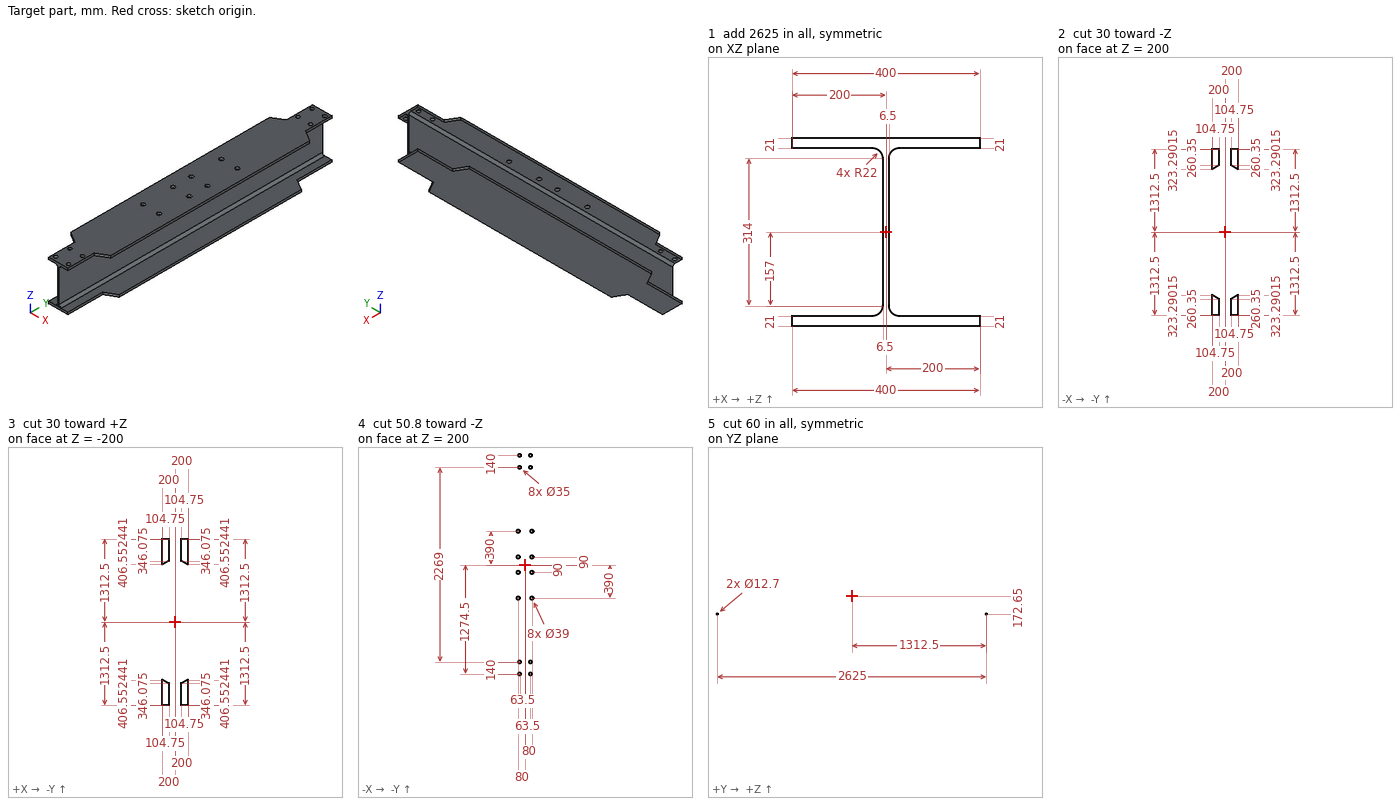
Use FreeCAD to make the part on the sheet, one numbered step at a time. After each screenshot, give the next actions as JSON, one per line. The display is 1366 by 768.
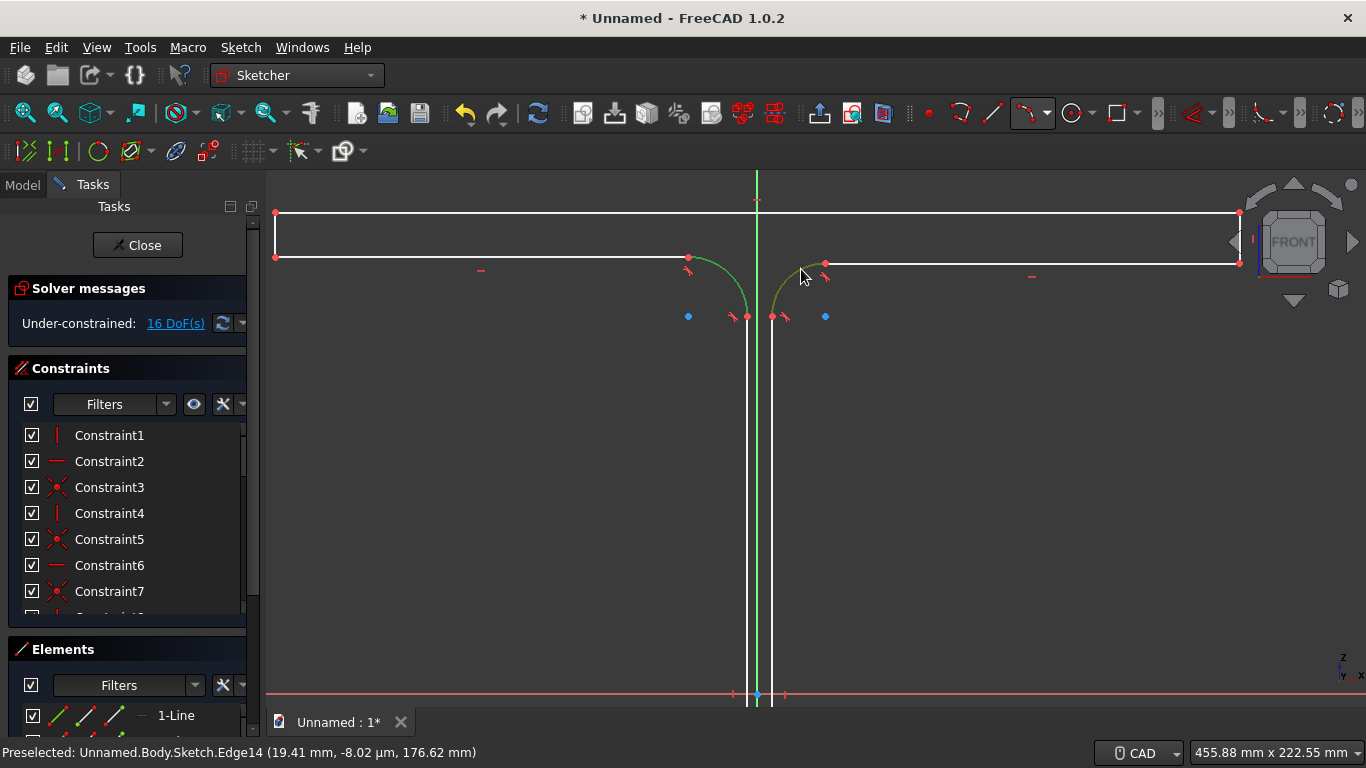
{"action": "scroll", "coordinate": [742, 290], "scroll_direction": "down", "scroll_amount": 5}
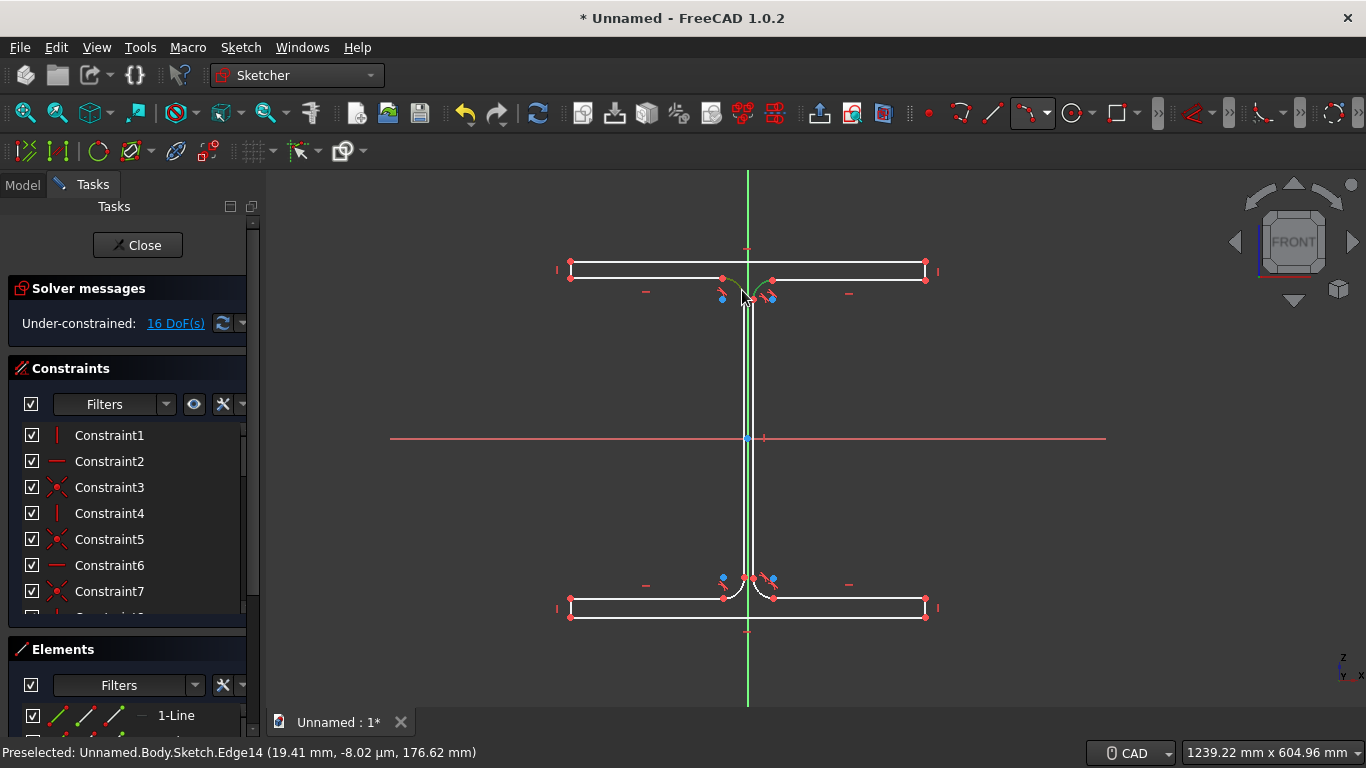
{"action": "scroll", "coordinate": [756, 587], "scroll_direction": "up", "scroll_amount": 3}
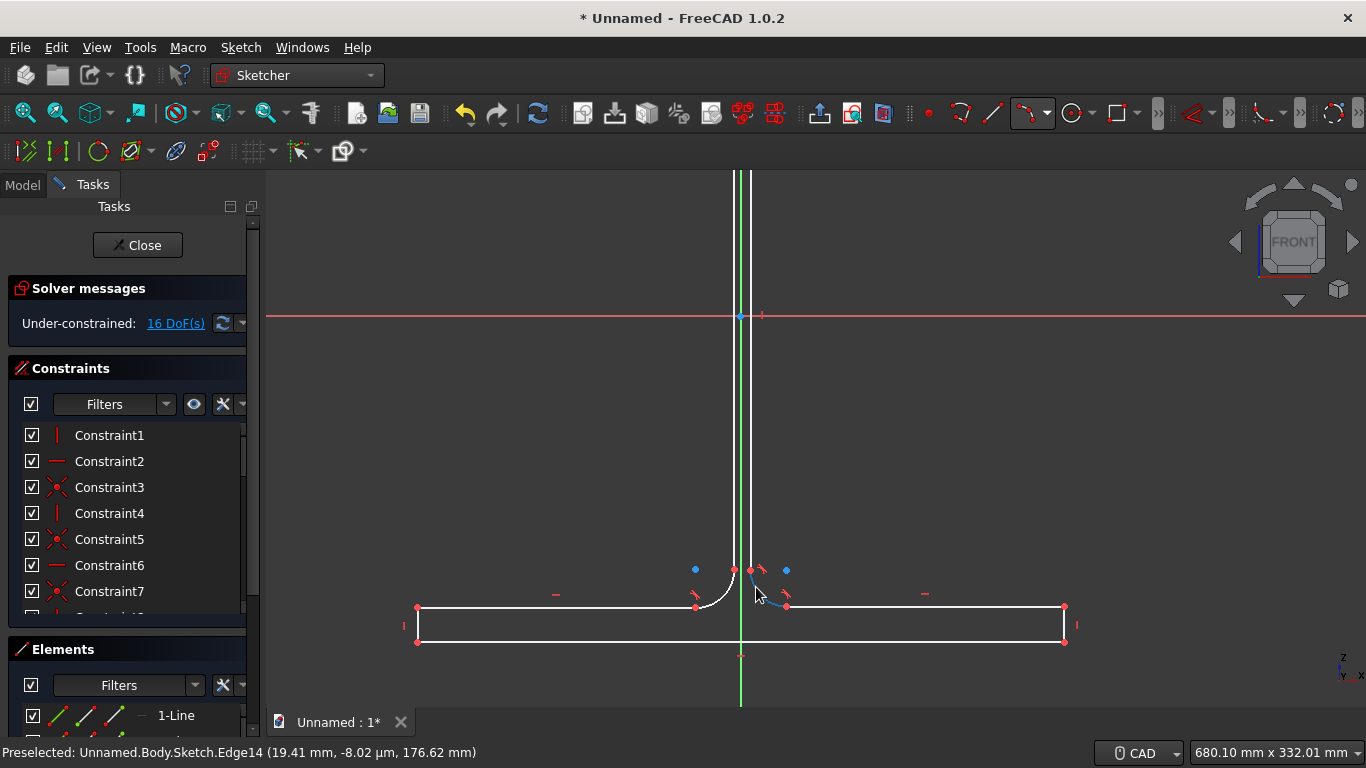
{"action": "left_click", "coordinate": [755, 587]}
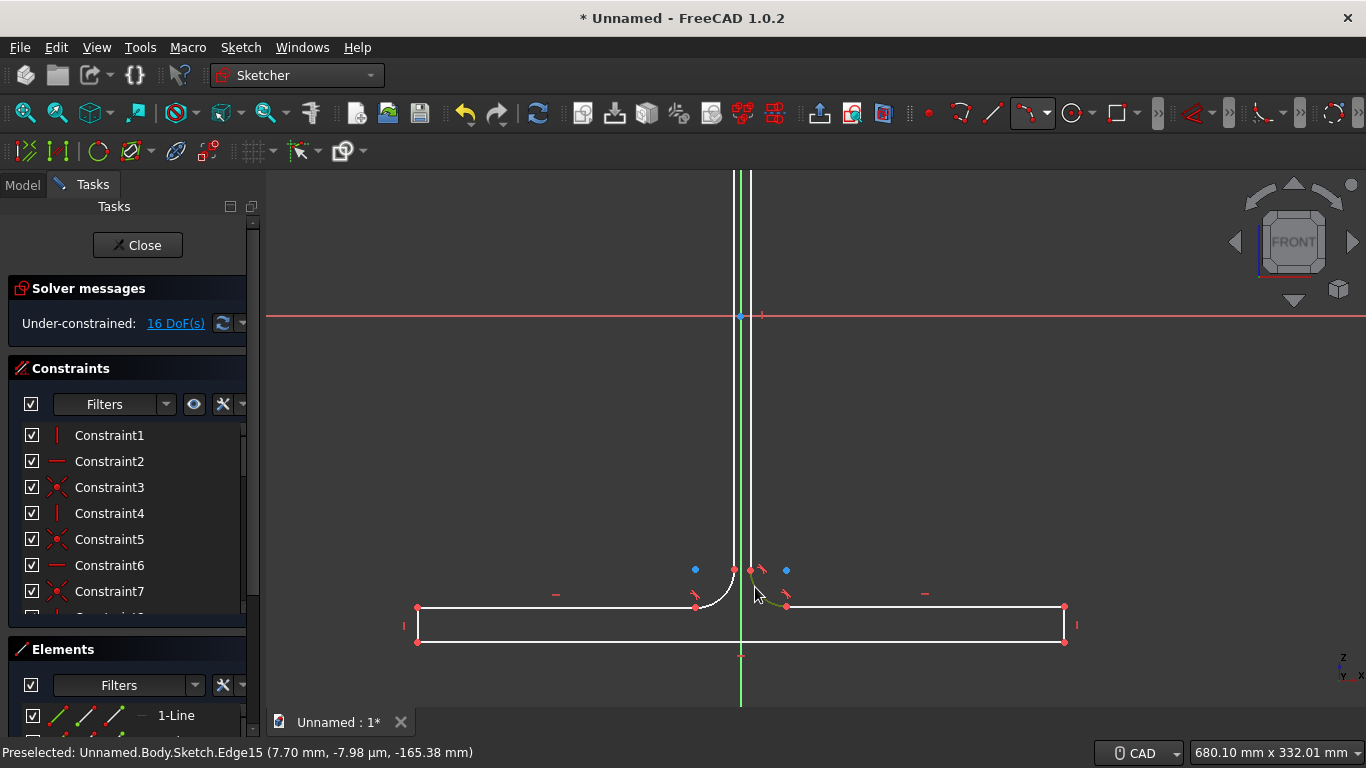
{"action": "left_click", "coordinate": [713, 604]}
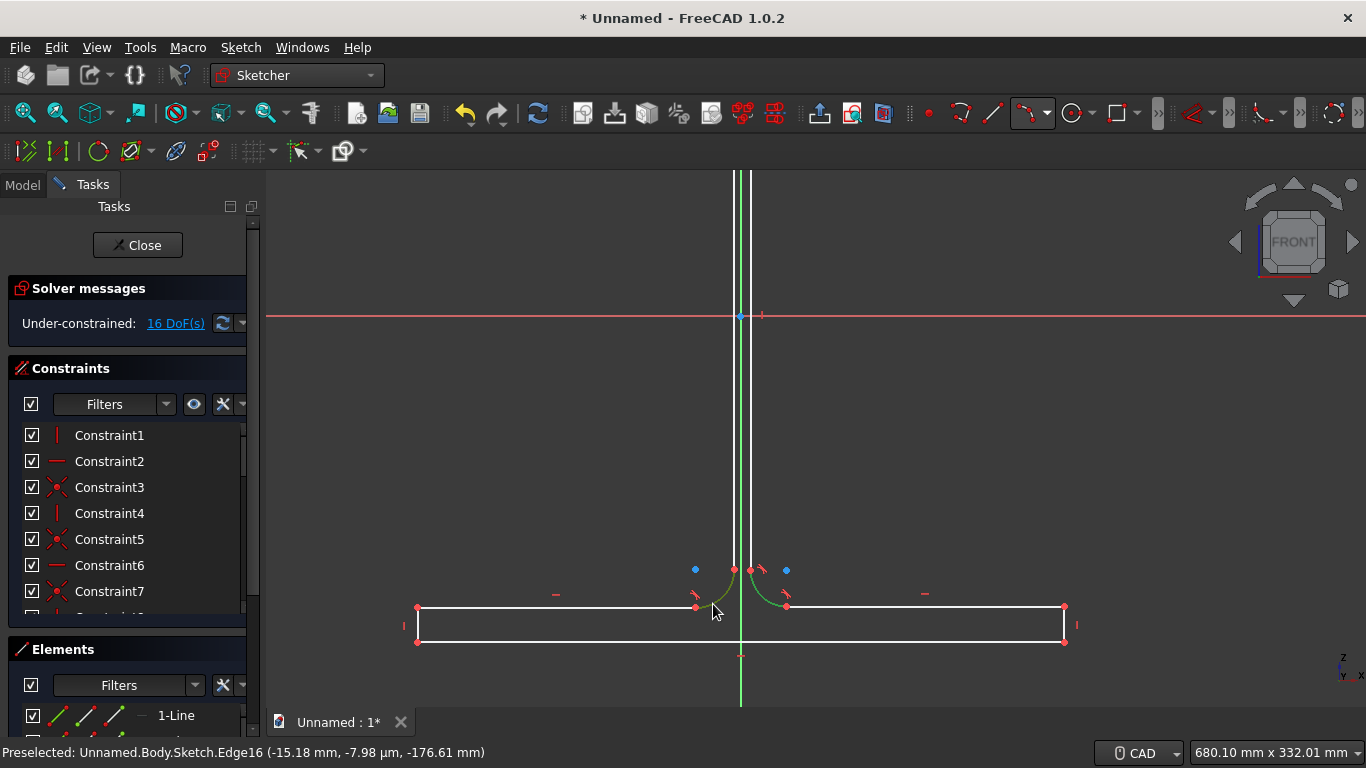
{"action": "key", "text": "e"}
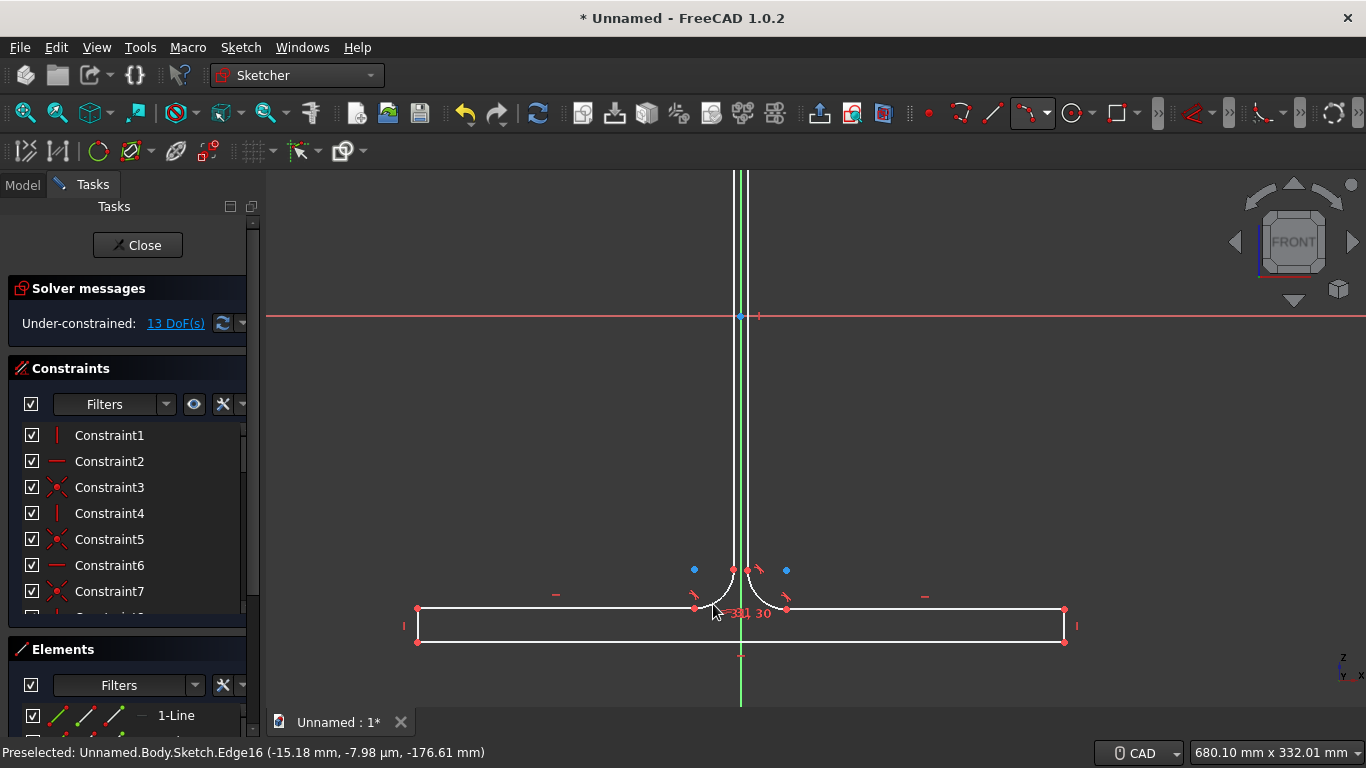
{"action": "left_click", "coordinate": [1192, 114]}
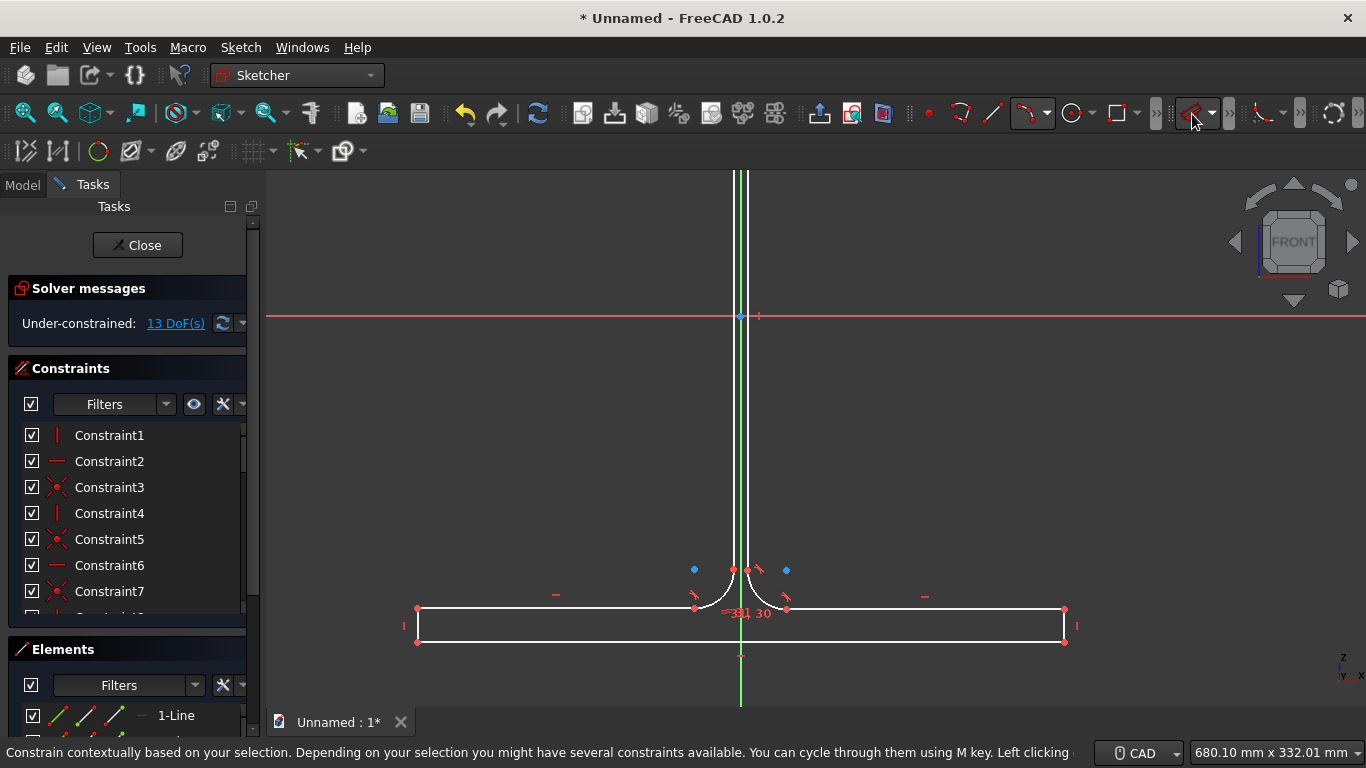
{"action": "scroll", "coordinate": [756, 587], "scroll_direction": "down", "scroll_amount": 3}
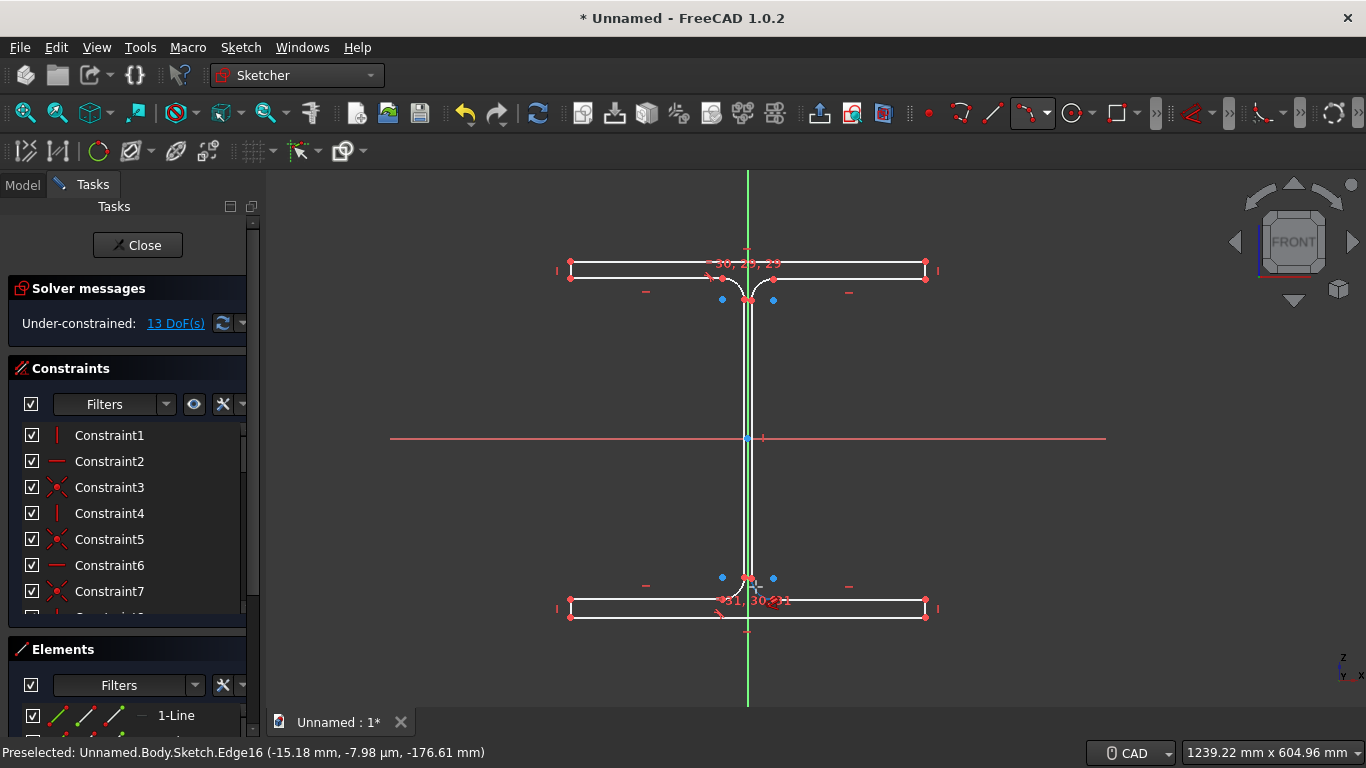
{"action": "scroll", "coordinate": [742, 290], "scroll_direction": "up", "scroll_amount": 5}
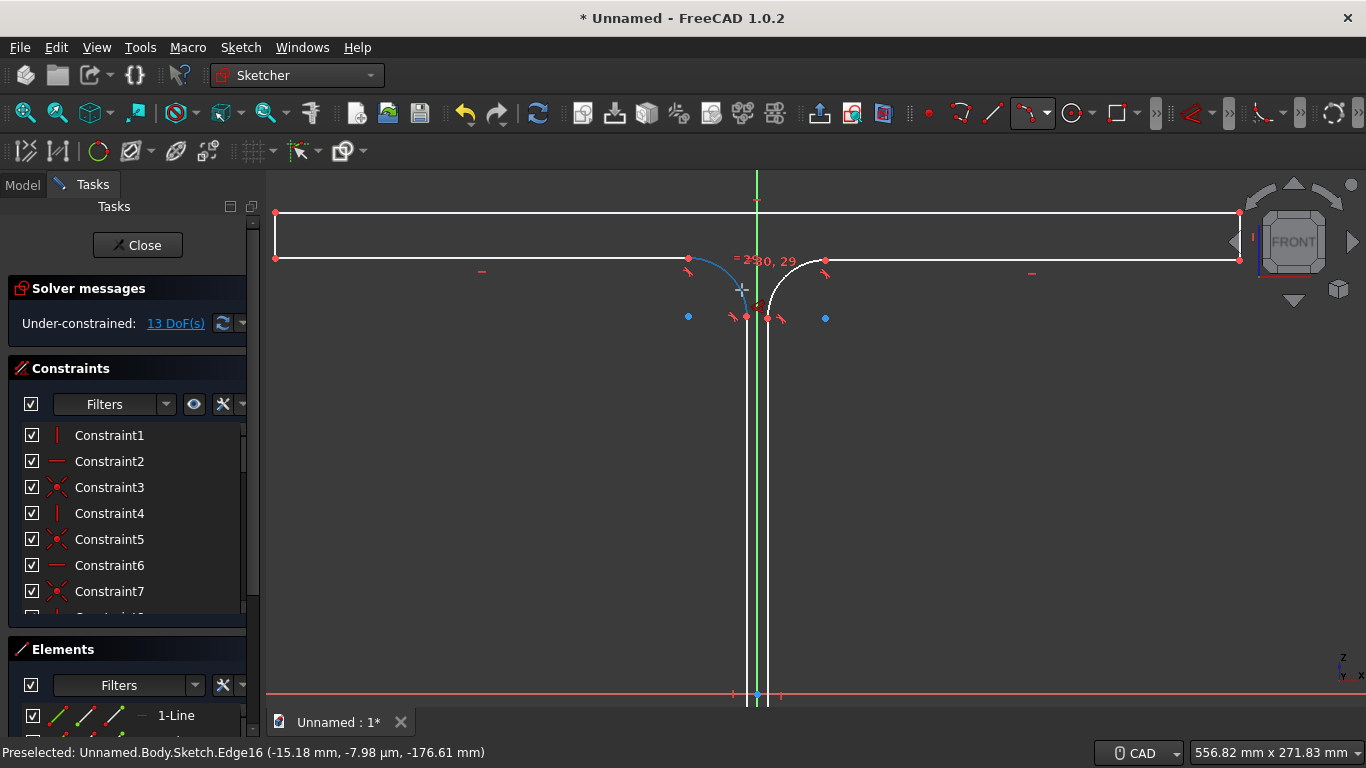
{"action": "left_click", "coordinate": [741, 290]}
{"action": "left_click", "coordinate": [740, 242]}